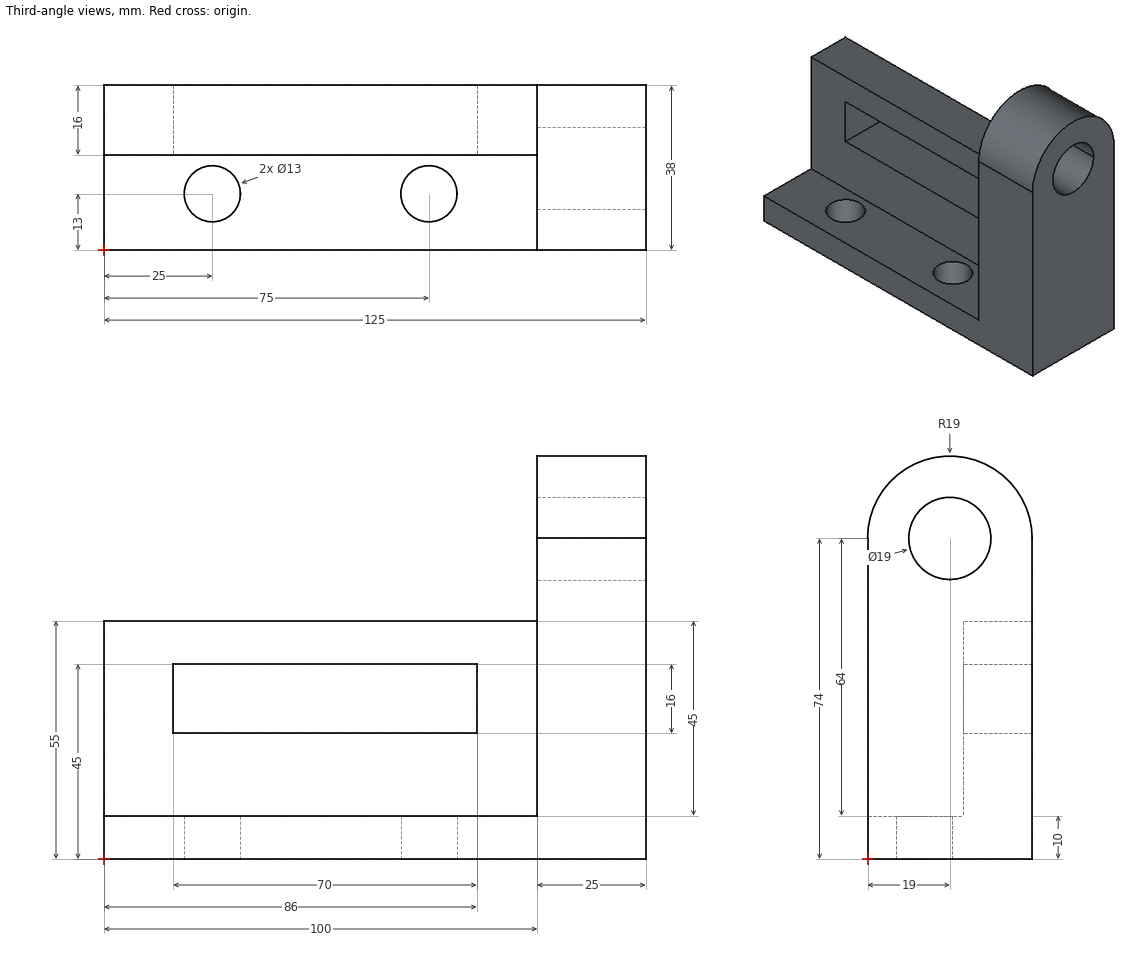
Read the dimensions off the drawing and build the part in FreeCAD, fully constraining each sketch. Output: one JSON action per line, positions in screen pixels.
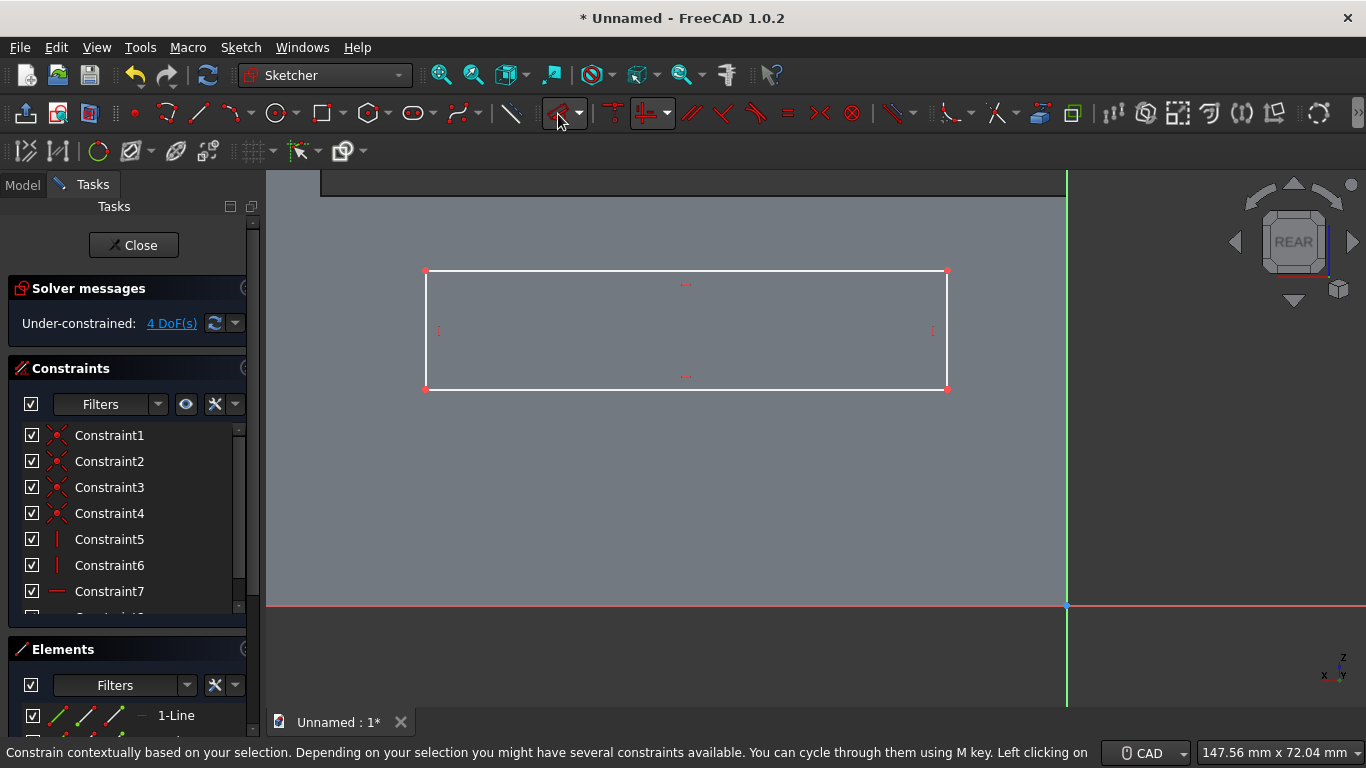
{"action": "left_click", "coordinate": [426, 307]}
{"action": "left_click", "coordinate": [392, 330]}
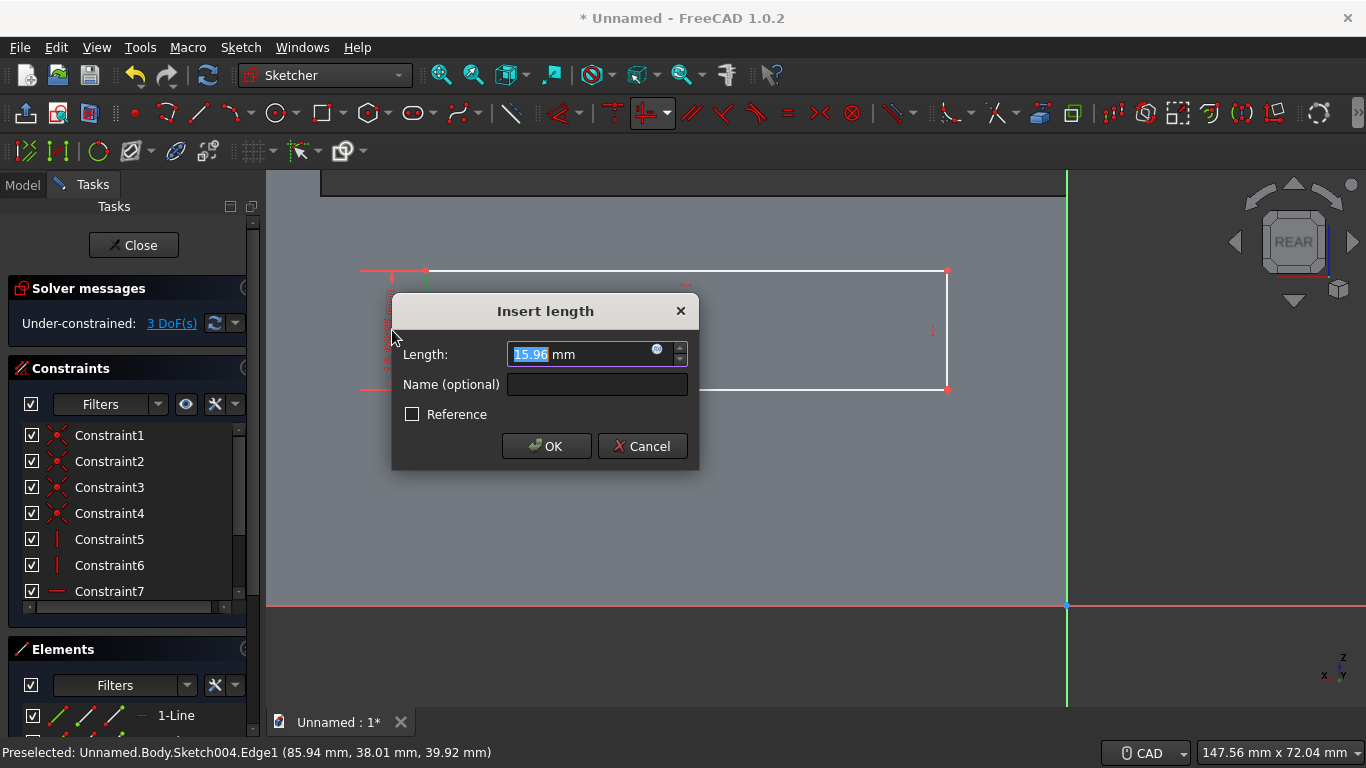
{"action": "type", "text": "16"}
{"action": "key", "text": "Return"}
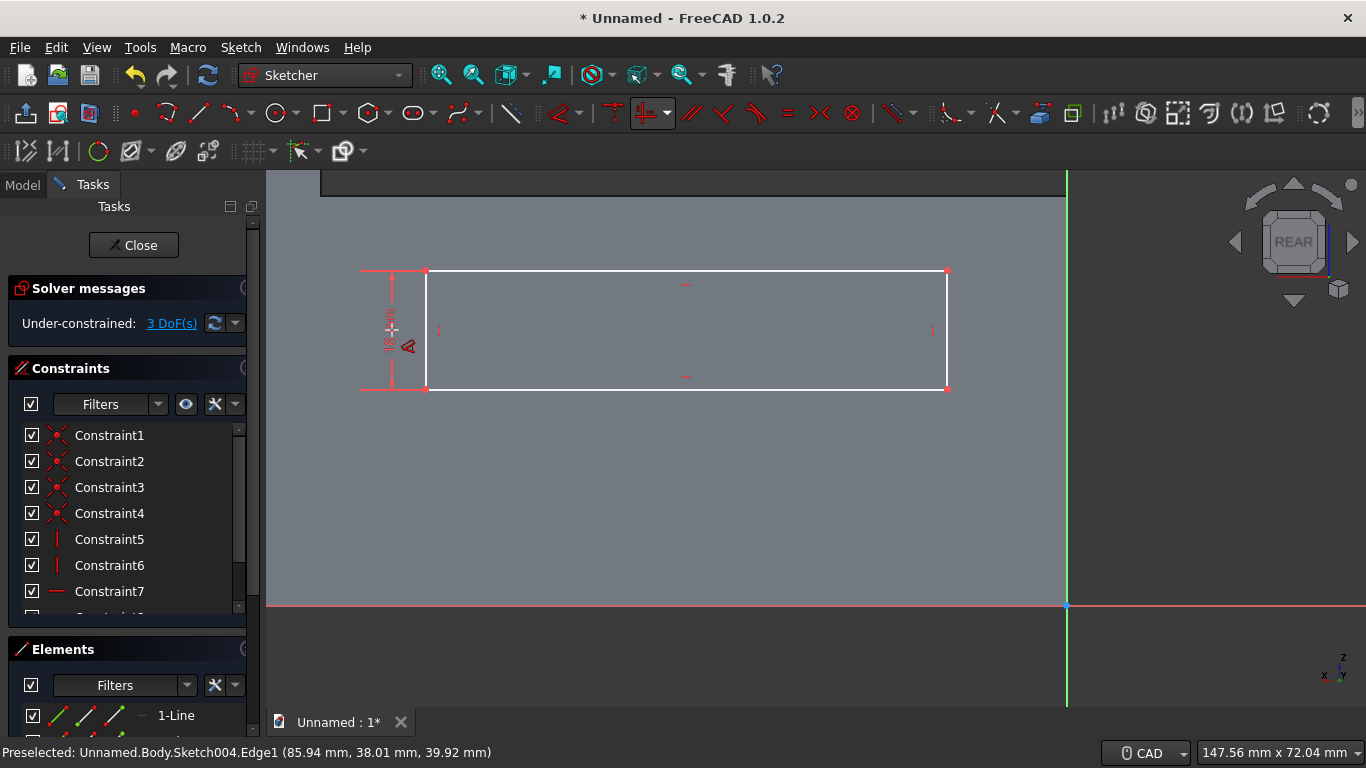
{"action": "left_click", "coordinate": [582, 390]}
{"action": "left_click", "coordinate": [687, 356]}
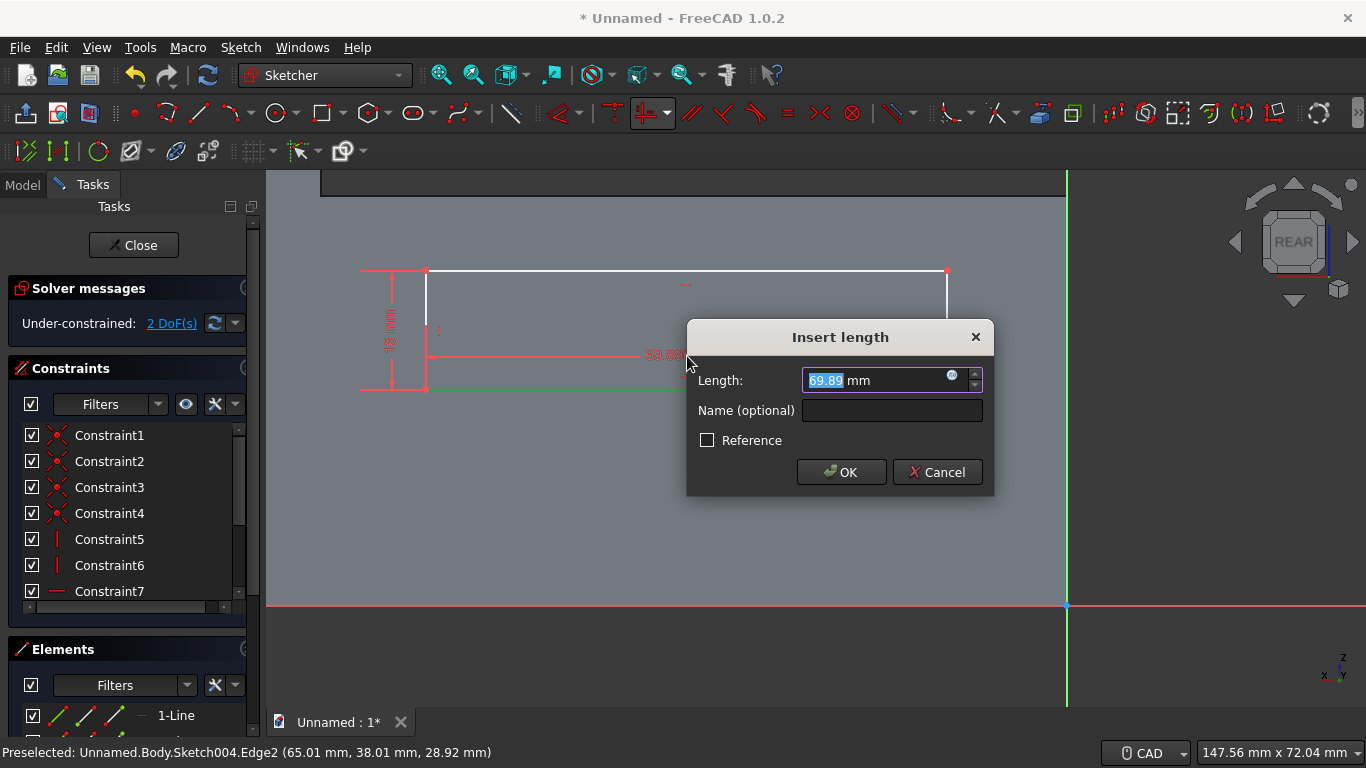
{"action": "type", "text": "70"}
{"action": "key", "text": "Return"}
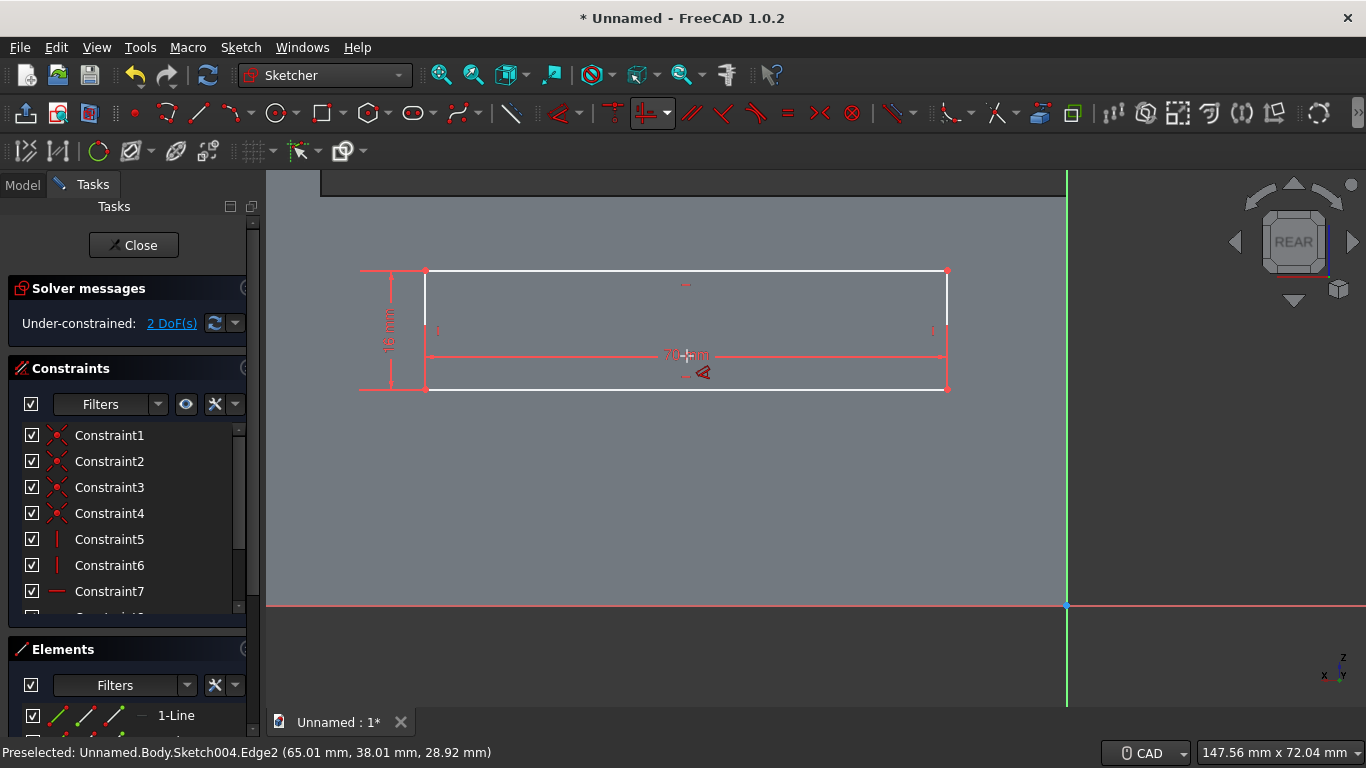
{"action": "left_click", "coordinate": [425, 271]}
{"action": "left_click", "coordinate": [746, 640]}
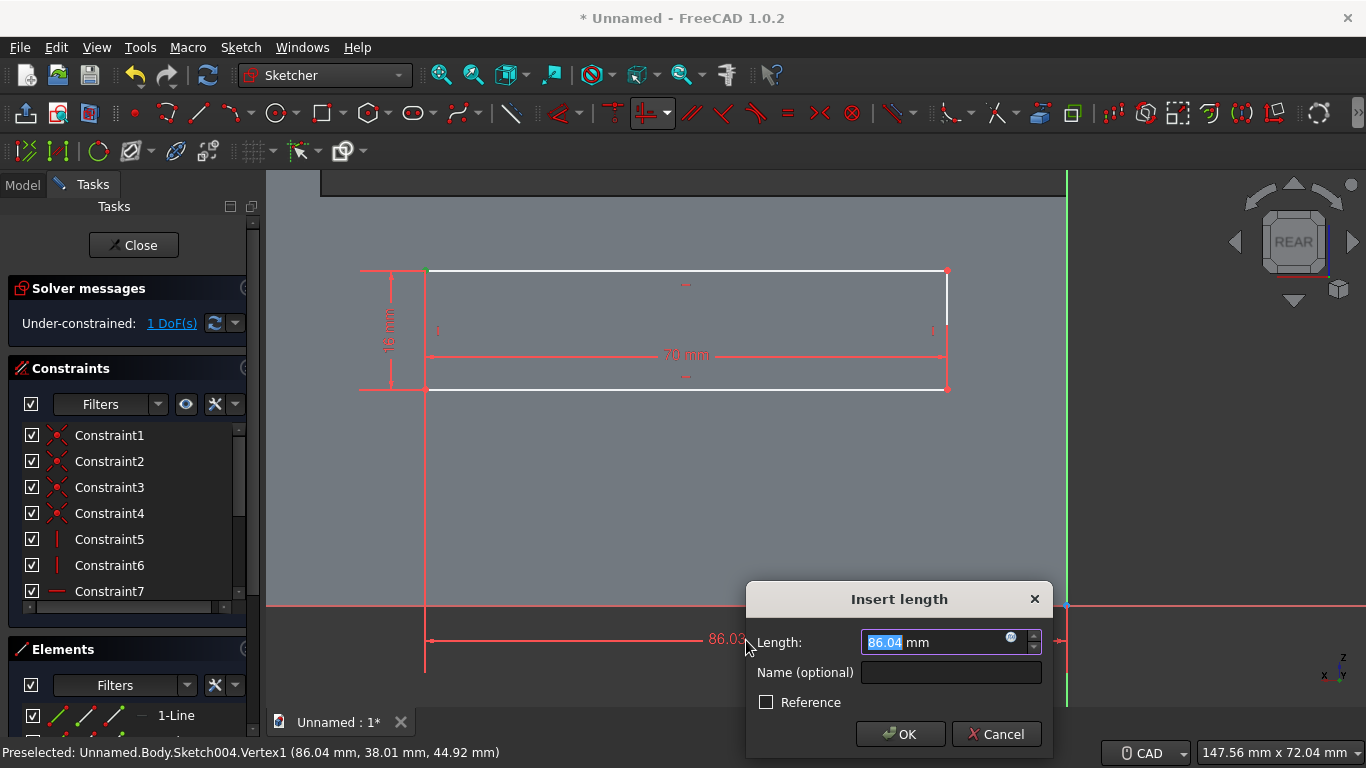
{"action": "type", "text": "86"}
{"action": "key", "text": "Return"}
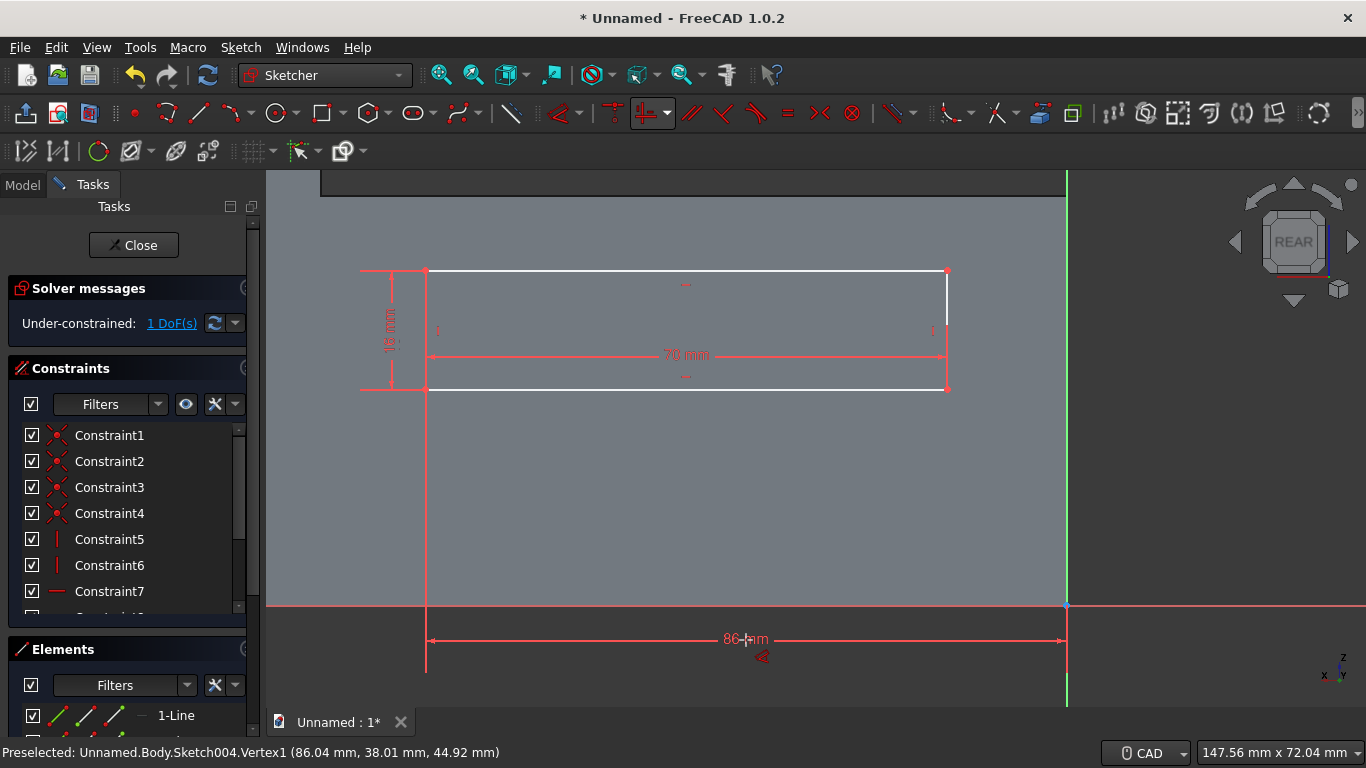
{"action": "left_click", "coordinate": [426, 271]}
{"action": "left_click", "coordinate": [1101, 438]}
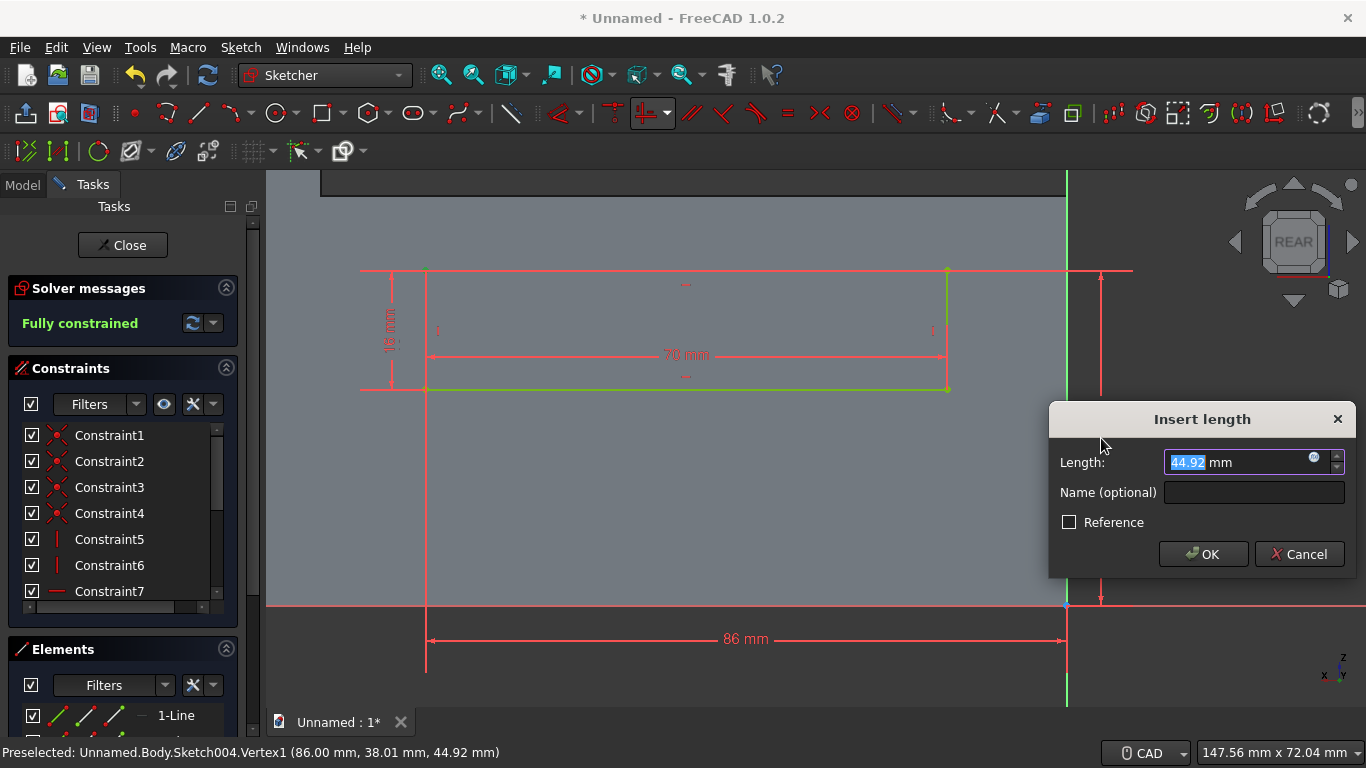
{"action": "type", "text": "45"}
{"action": "key", "text": "Return"}
{"action": "key", "text": "Escape"}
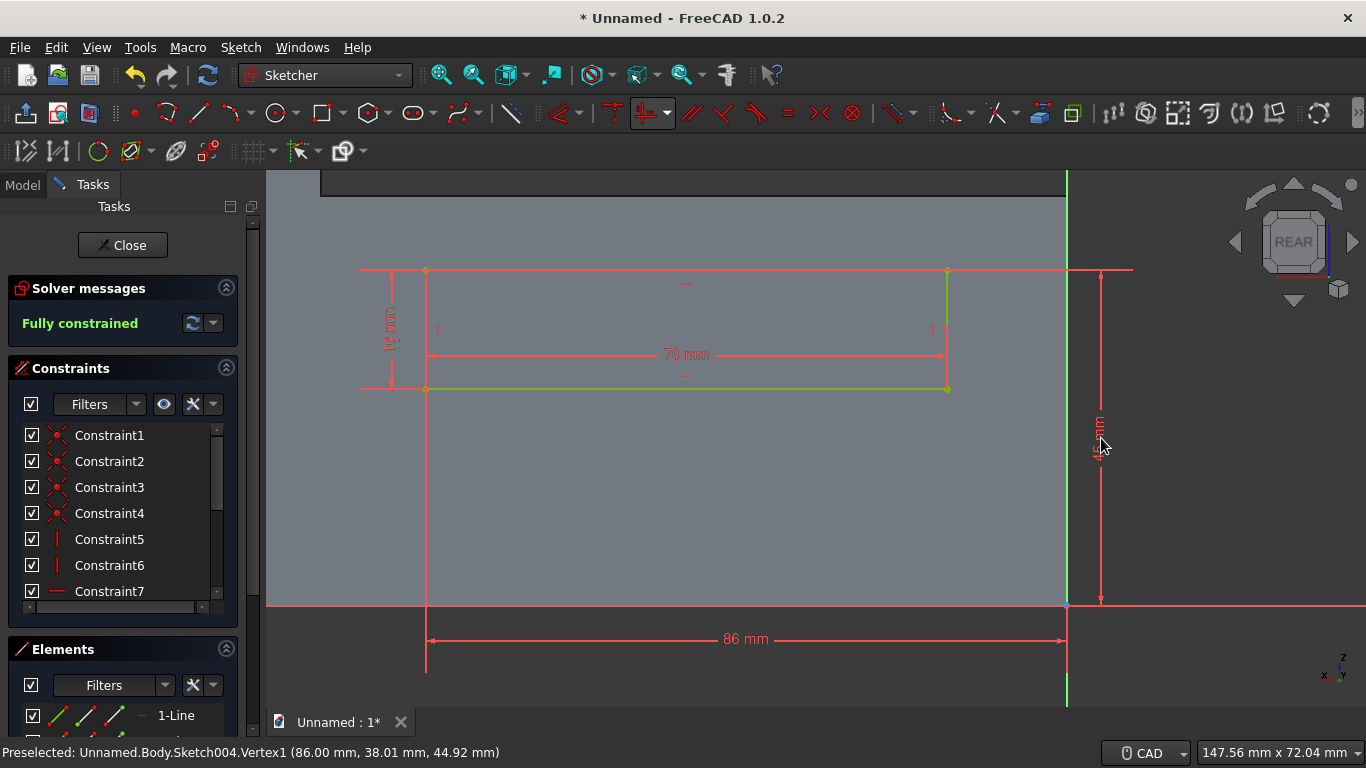
{"action": "left_click", "coordinate": [123, 245]}